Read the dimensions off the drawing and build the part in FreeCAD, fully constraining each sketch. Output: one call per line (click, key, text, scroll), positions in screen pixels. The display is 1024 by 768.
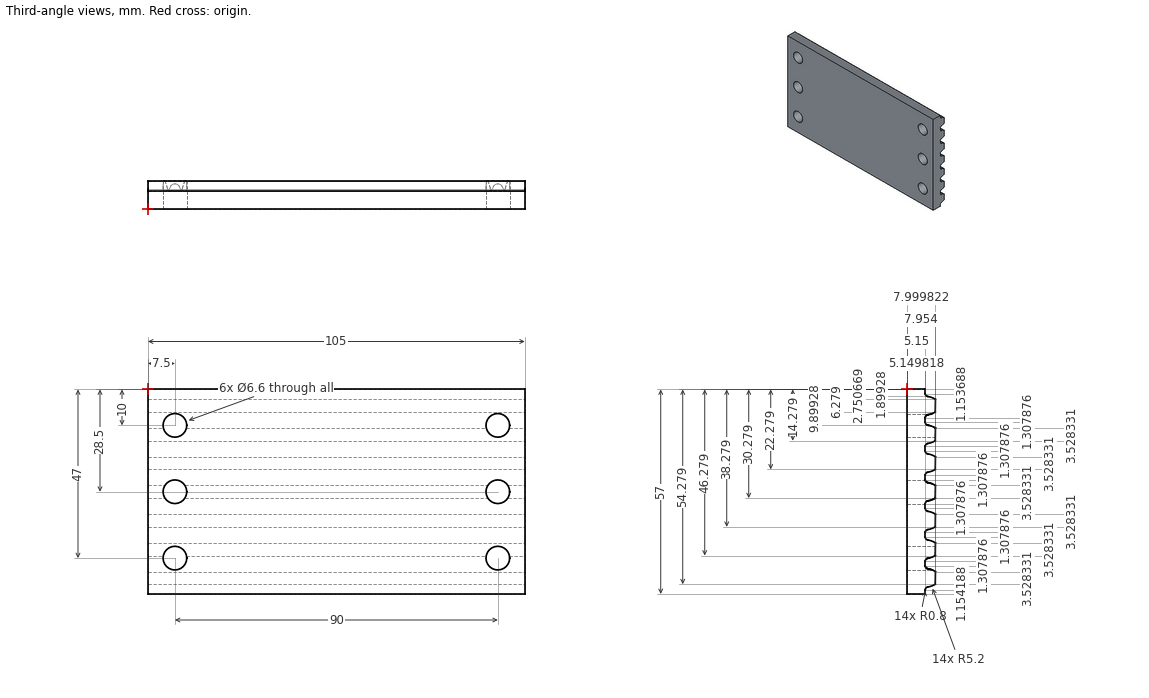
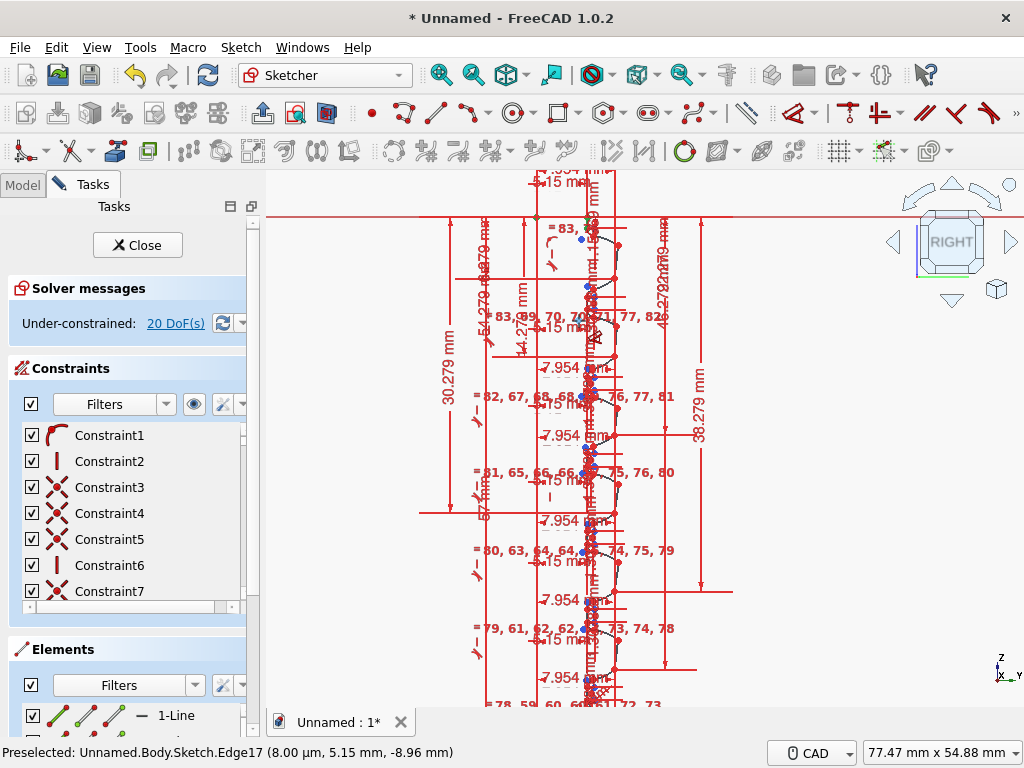
click(579, 321)
click(503, 269)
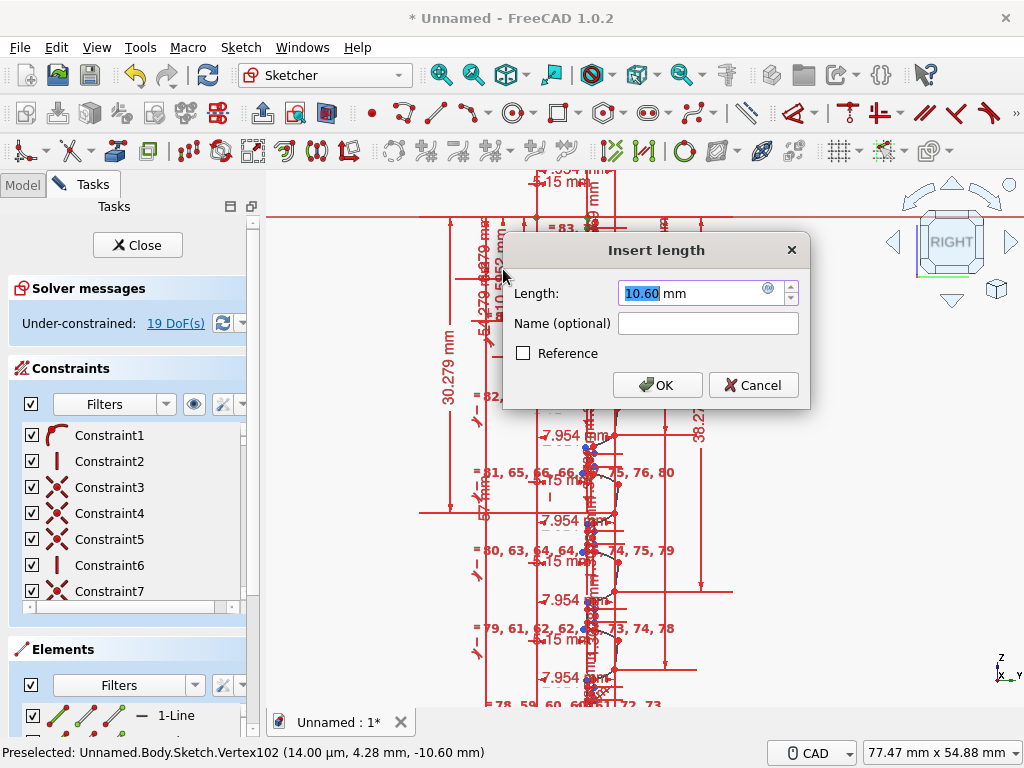
text(9.89928)
key(Return)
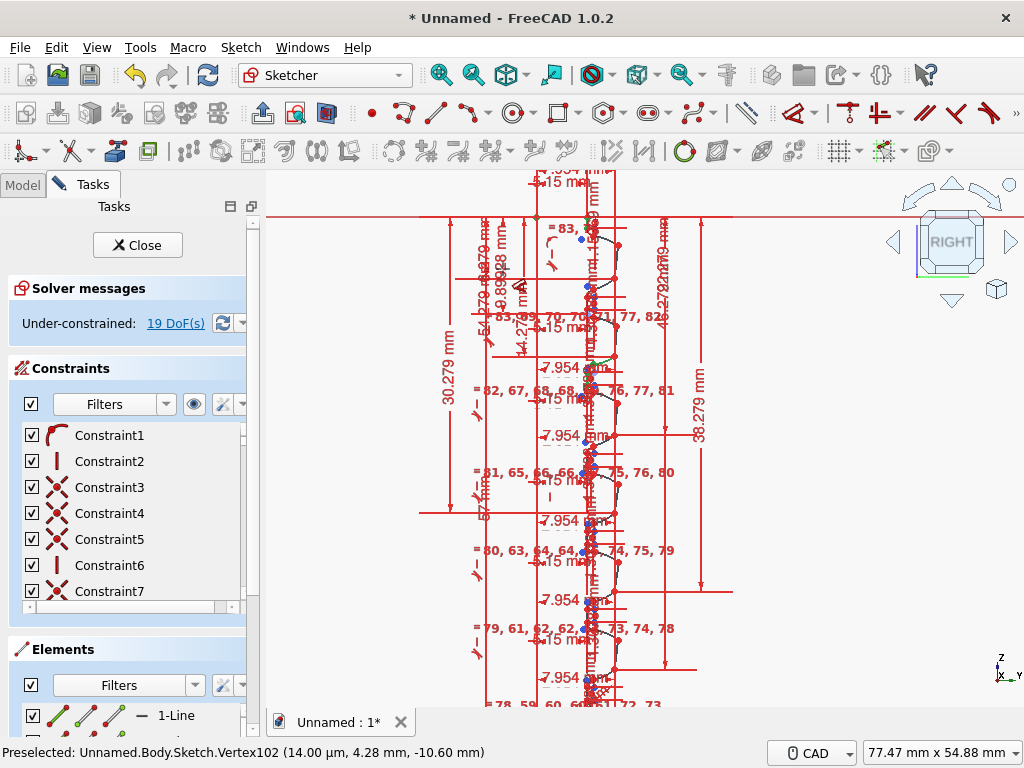
scroll(581, 240, up, 4)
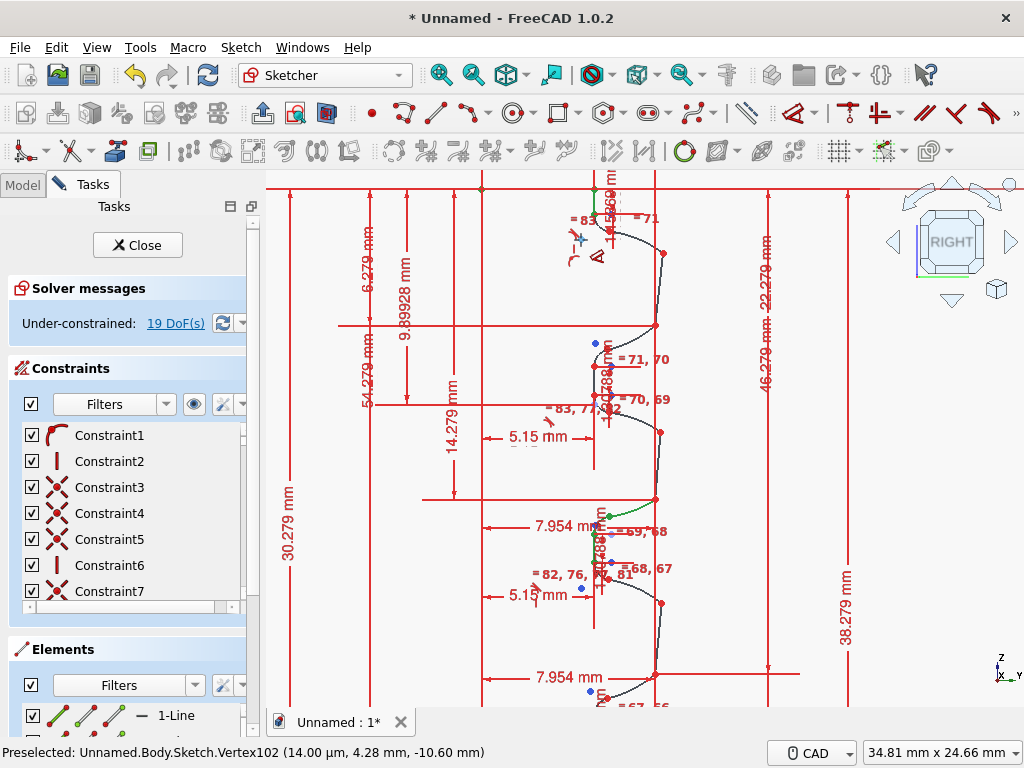
click(582, 240)
click(448, 219)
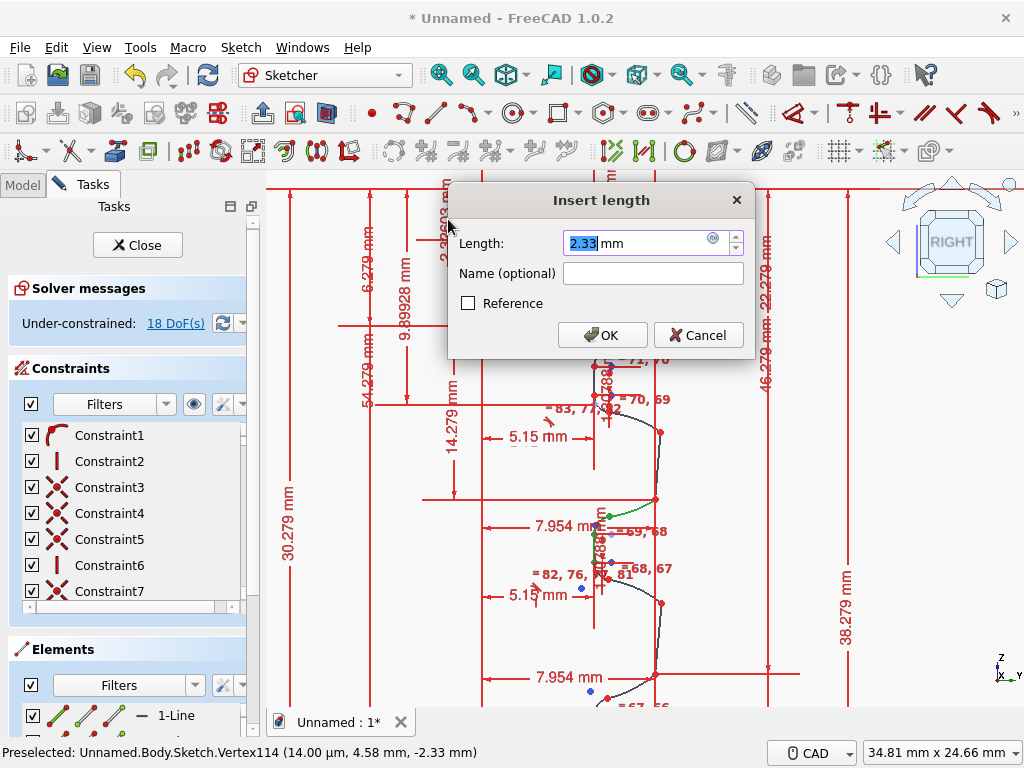
text(1.89928)
key(Return)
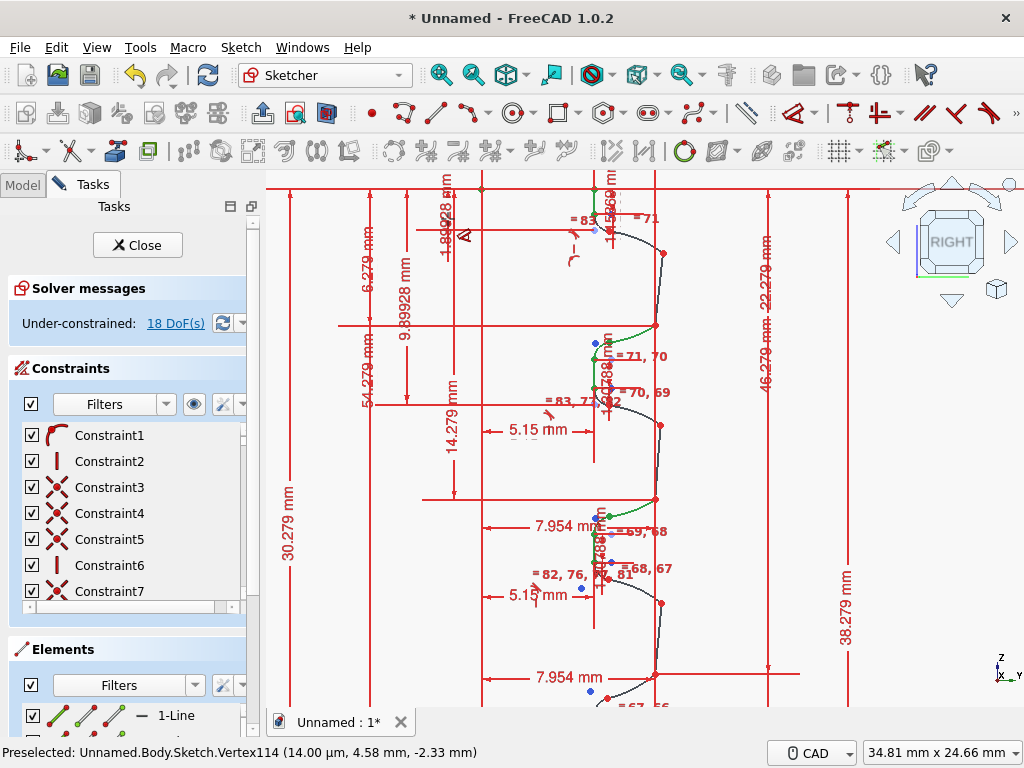
scroll(580, 279, down, 6)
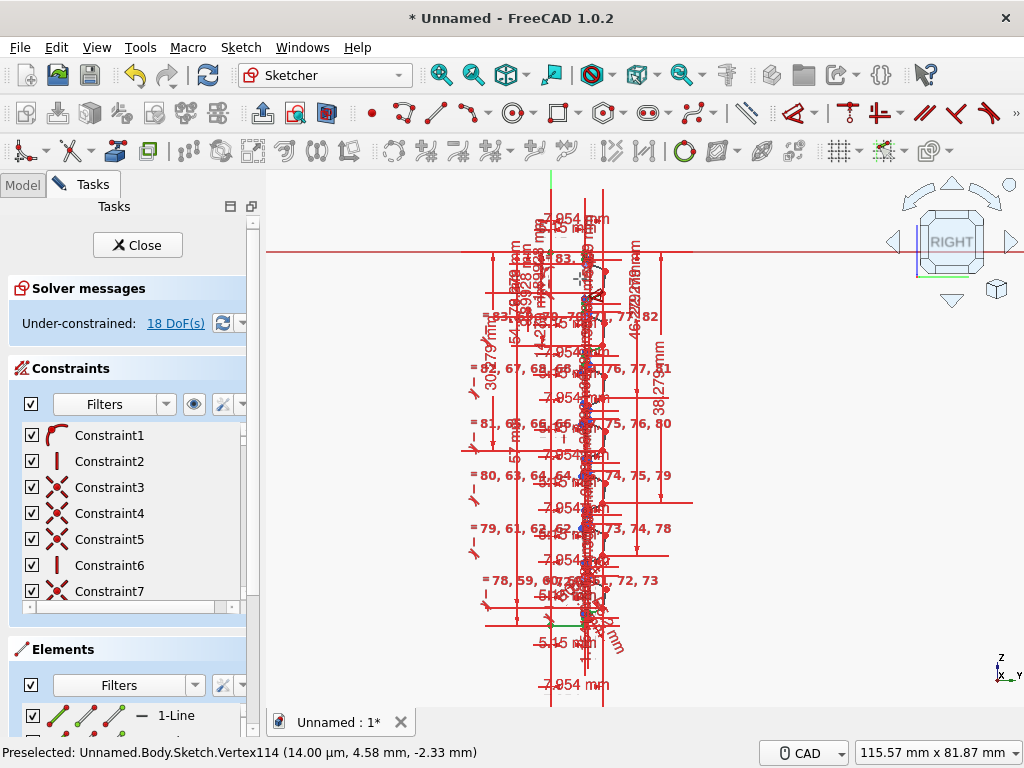
click(606, 589)
click(598, 647)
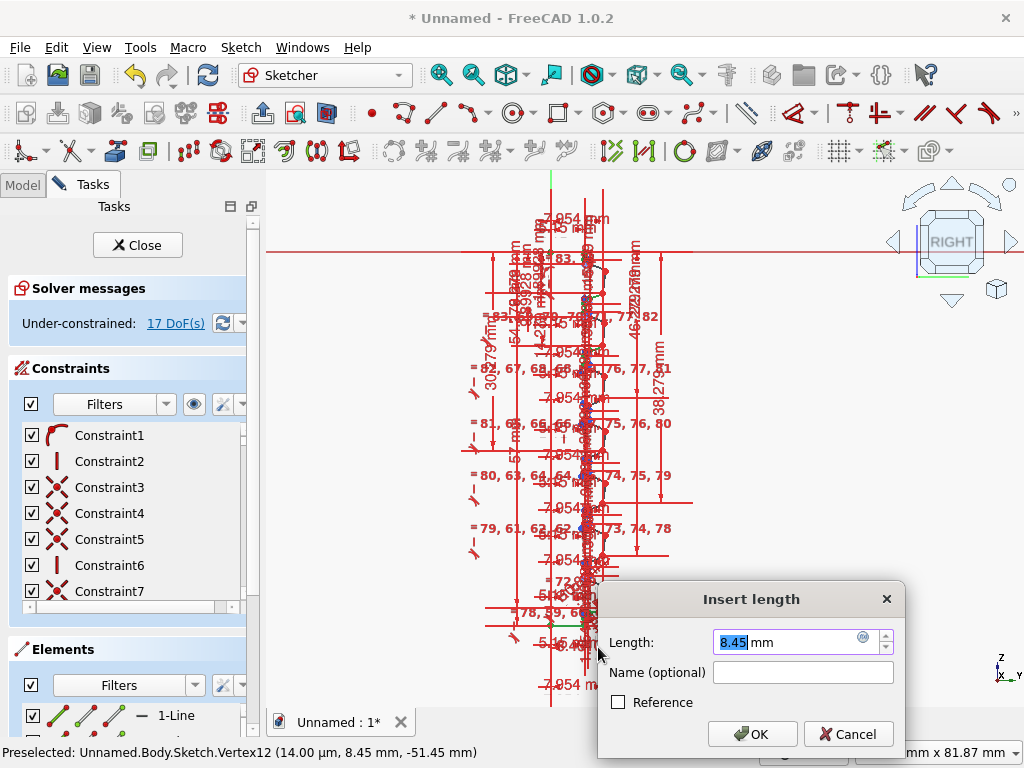
text(7.999822)
key(Return)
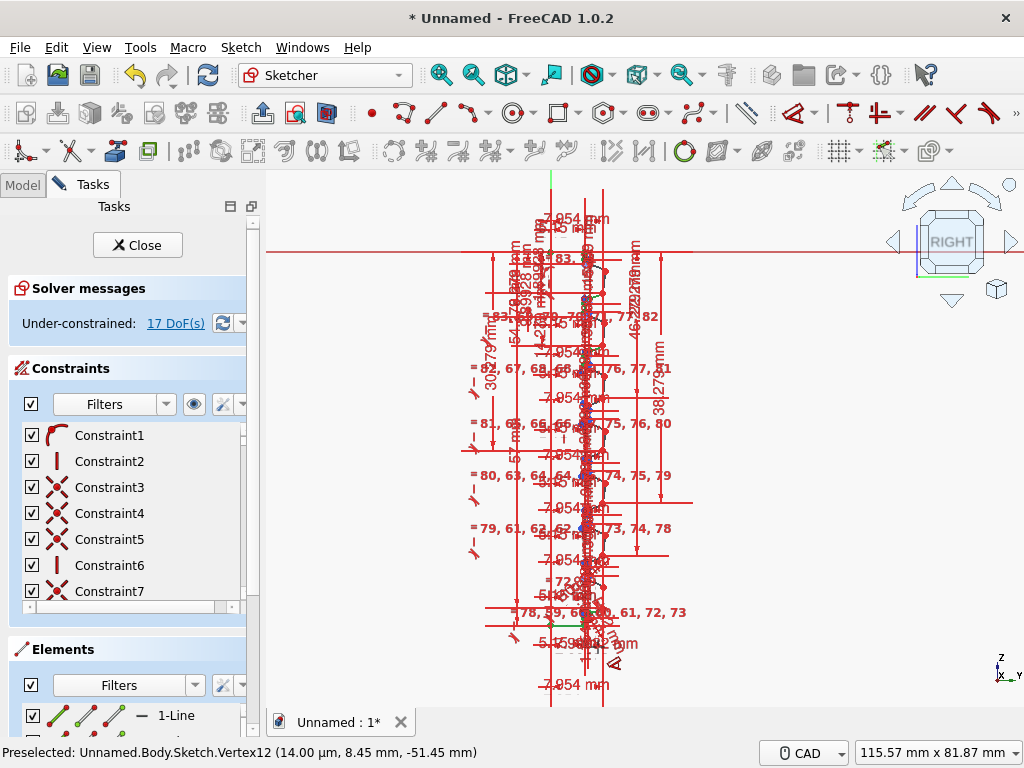
click(605, 536)
click(578, 666)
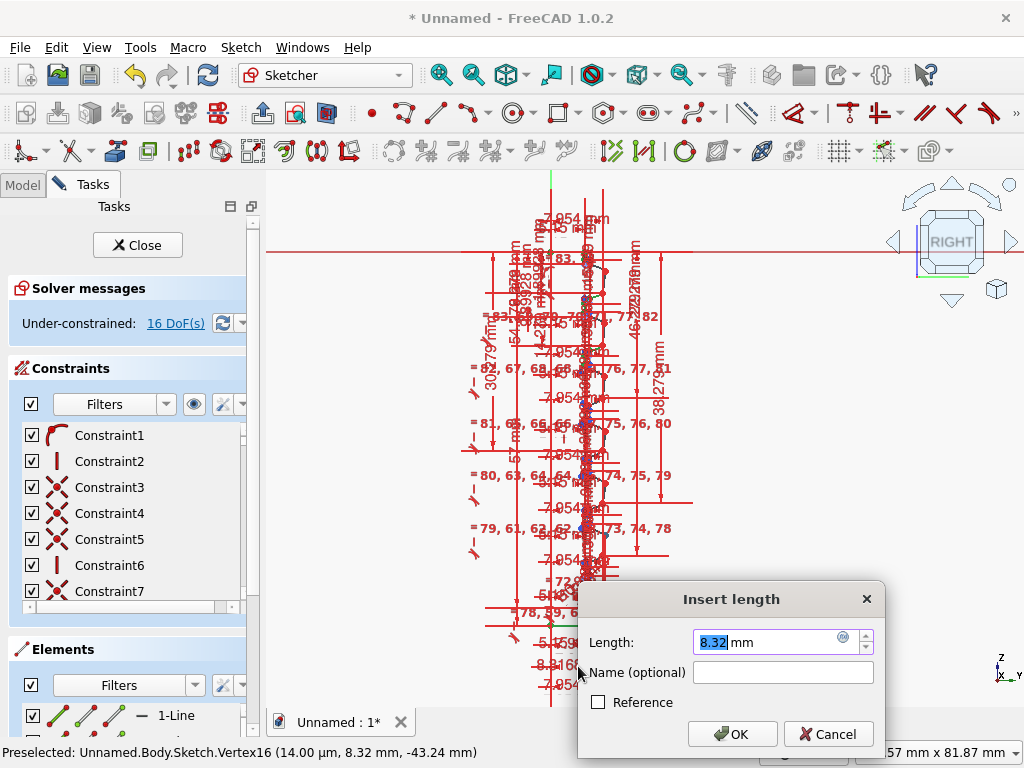
text(7.999822)
key(Return)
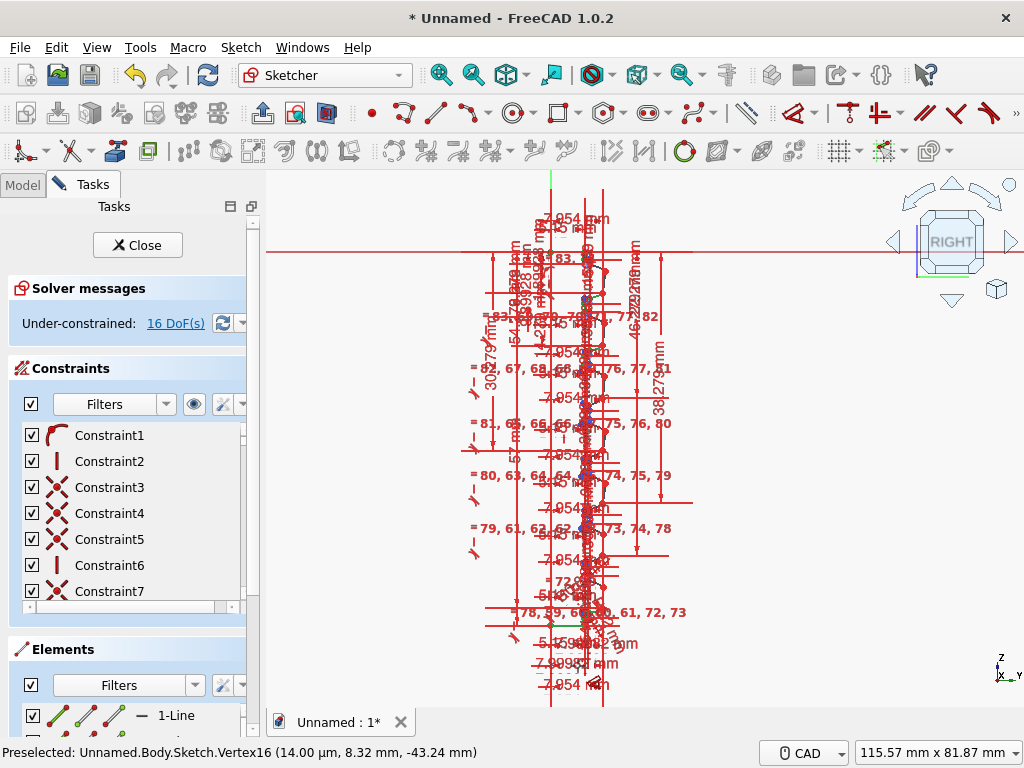
click(606, 484)
click(578, 218)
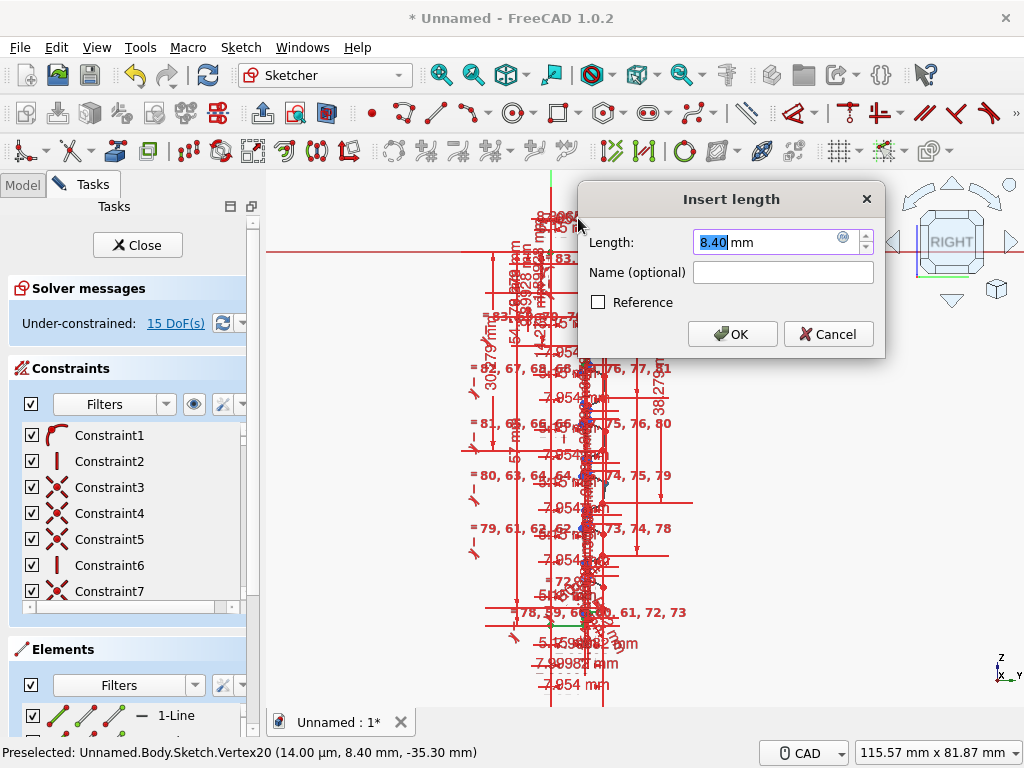
text(7.999822)
key(Return)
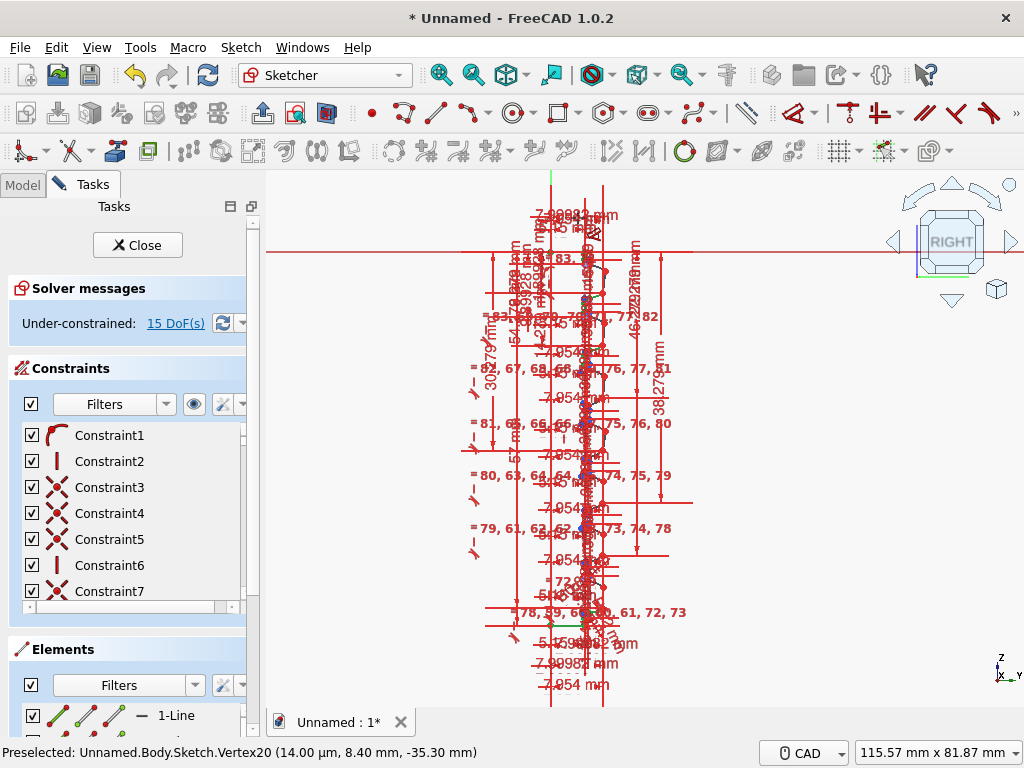
click(606, 431)
click(578, 218)